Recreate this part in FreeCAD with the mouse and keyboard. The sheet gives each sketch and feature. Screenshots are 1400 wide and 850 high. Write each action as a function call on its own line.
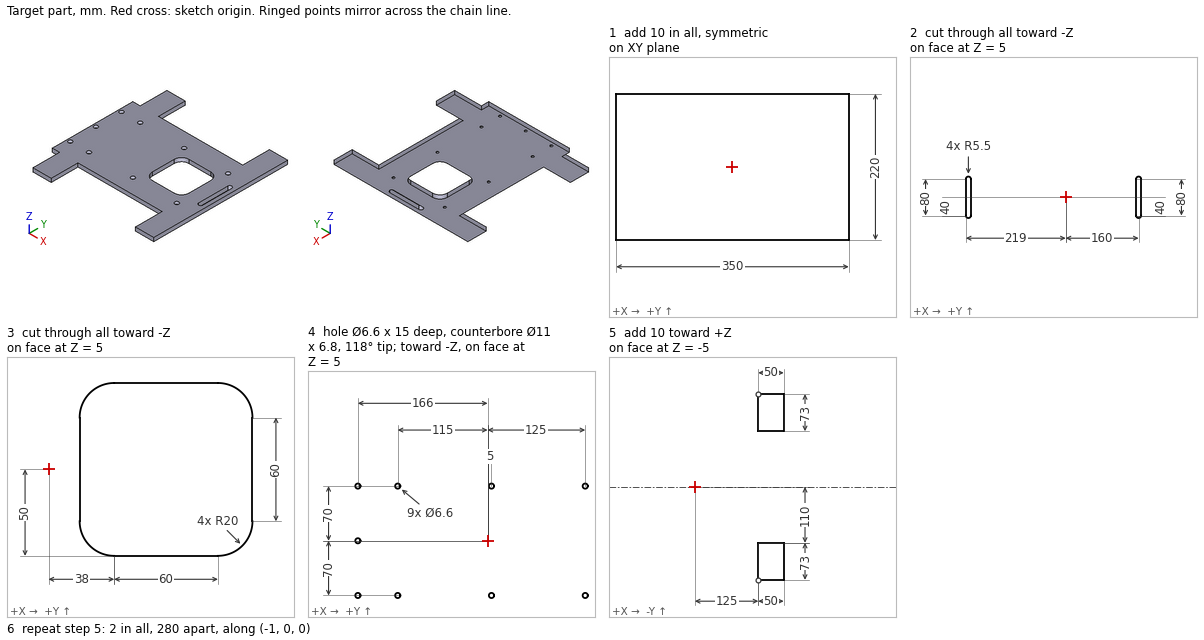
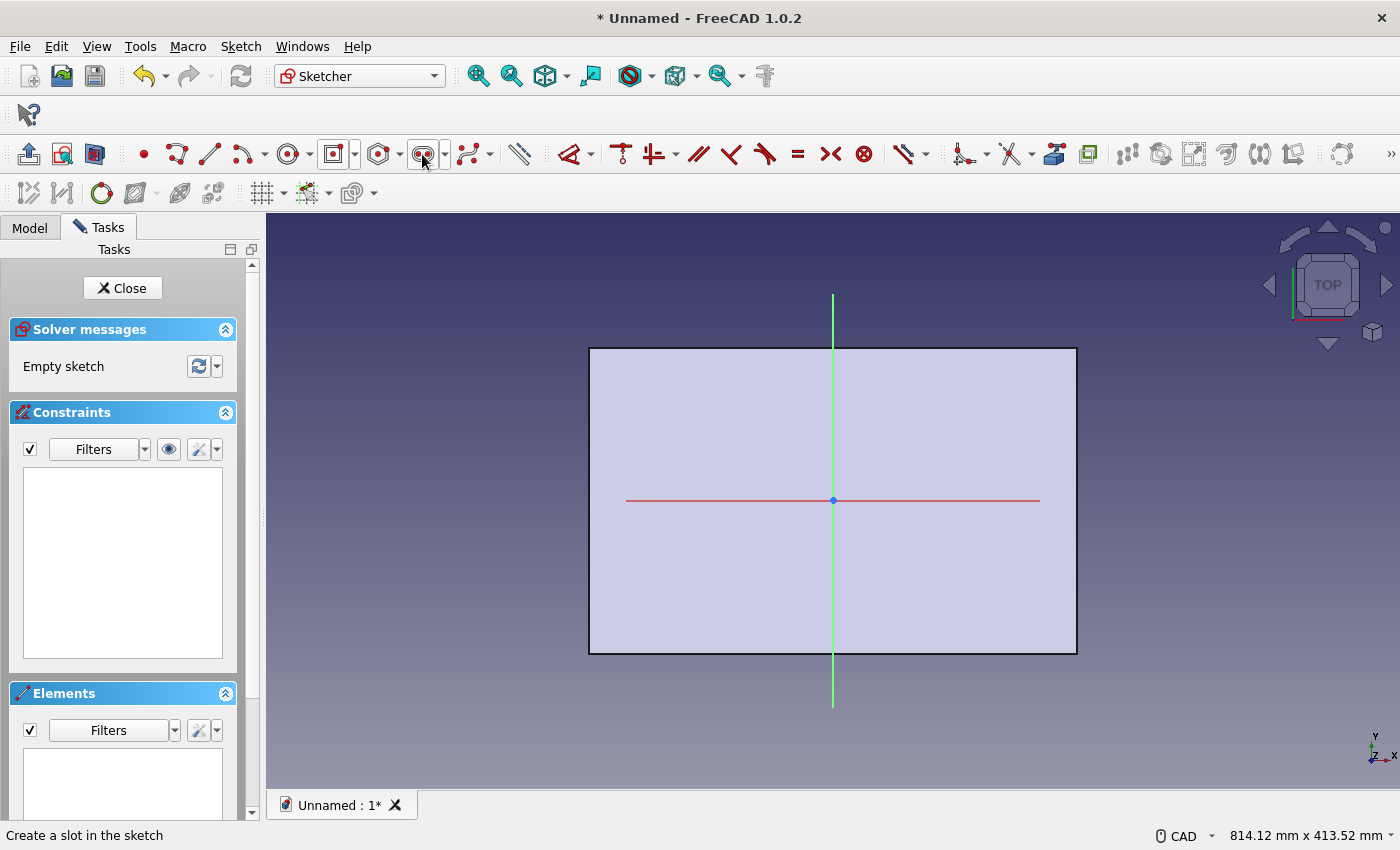
scroll(536, 557, up, 6)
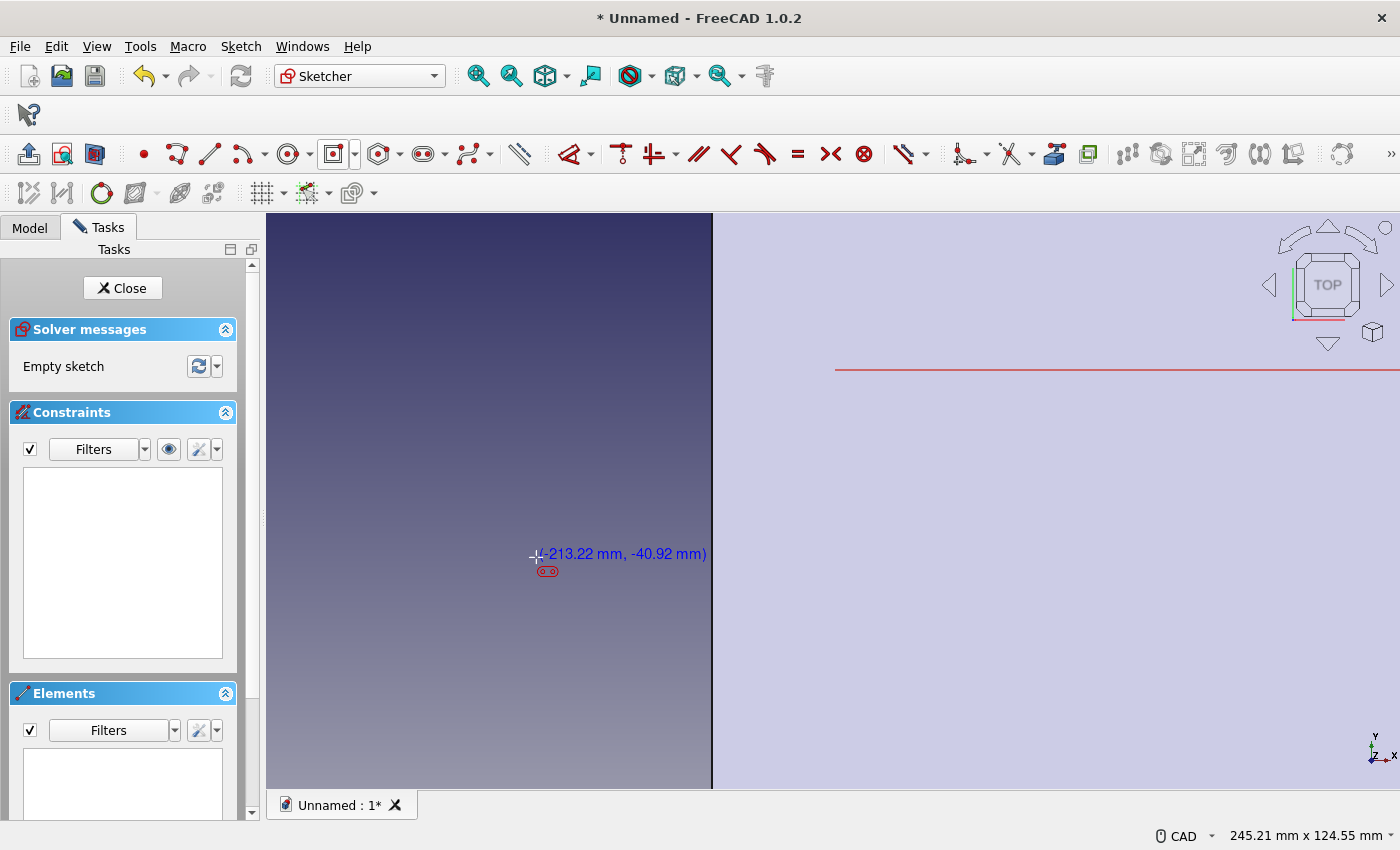
click(534, 555)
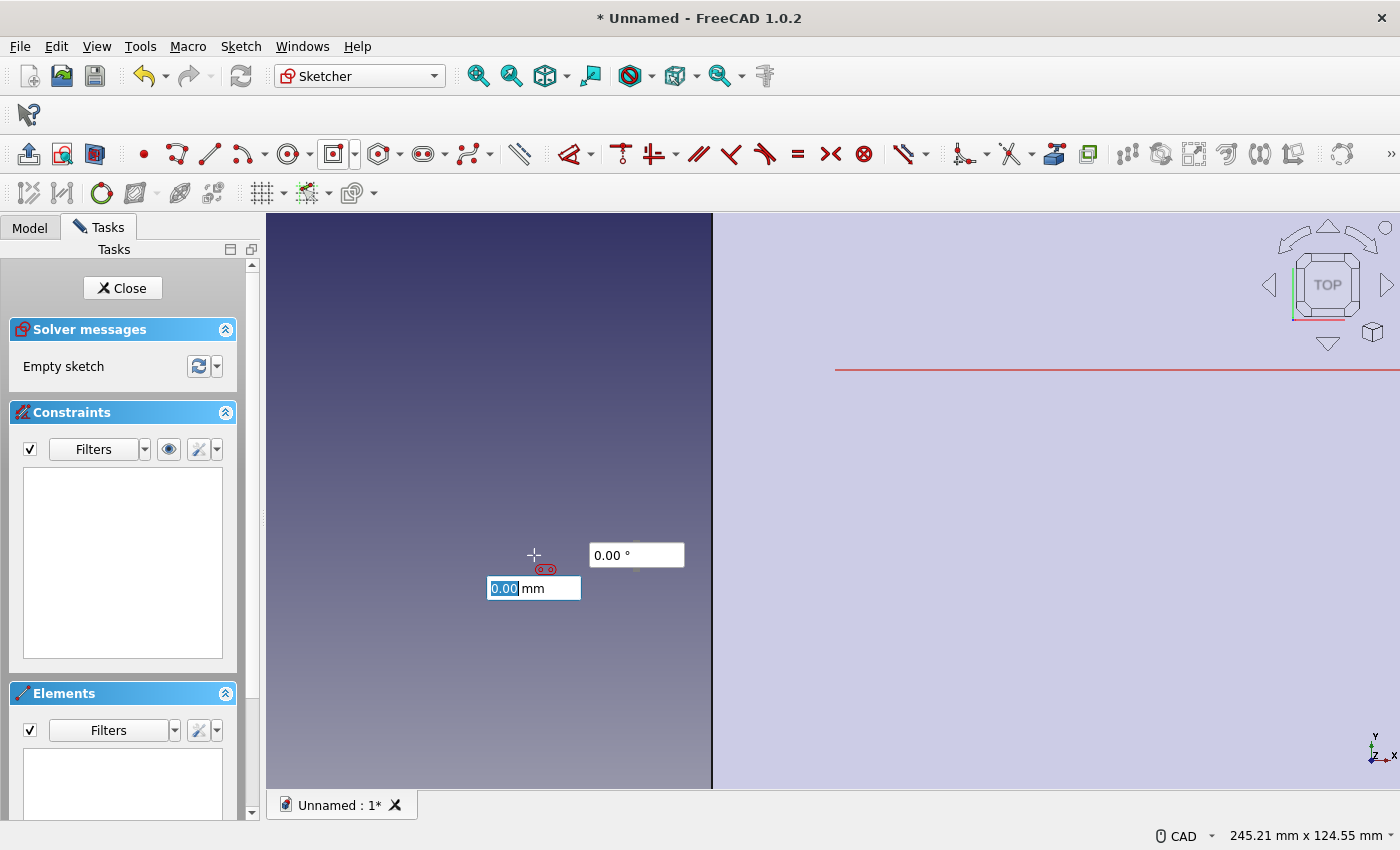
scroll(396, 577, down, 5)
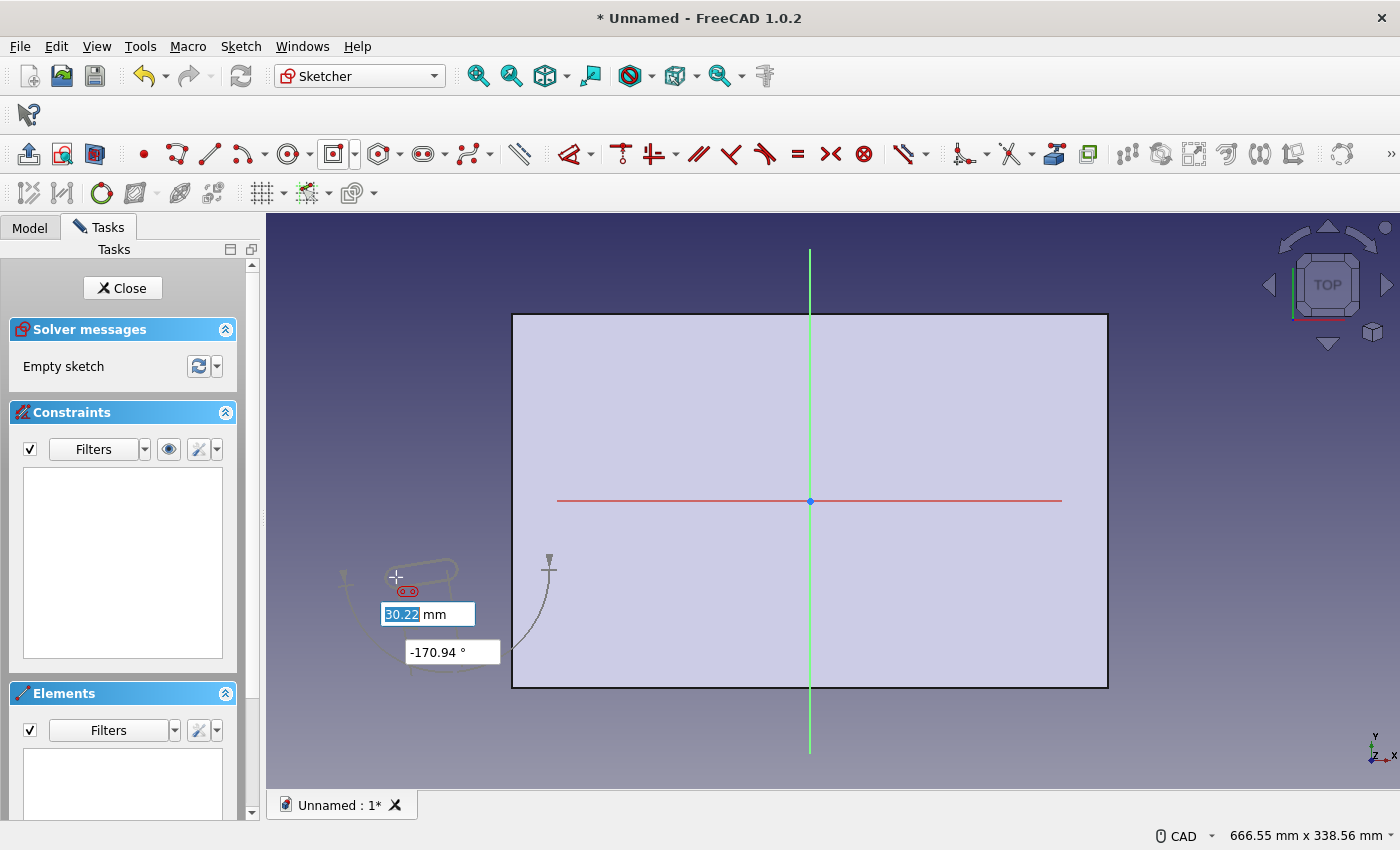
click(447, 433)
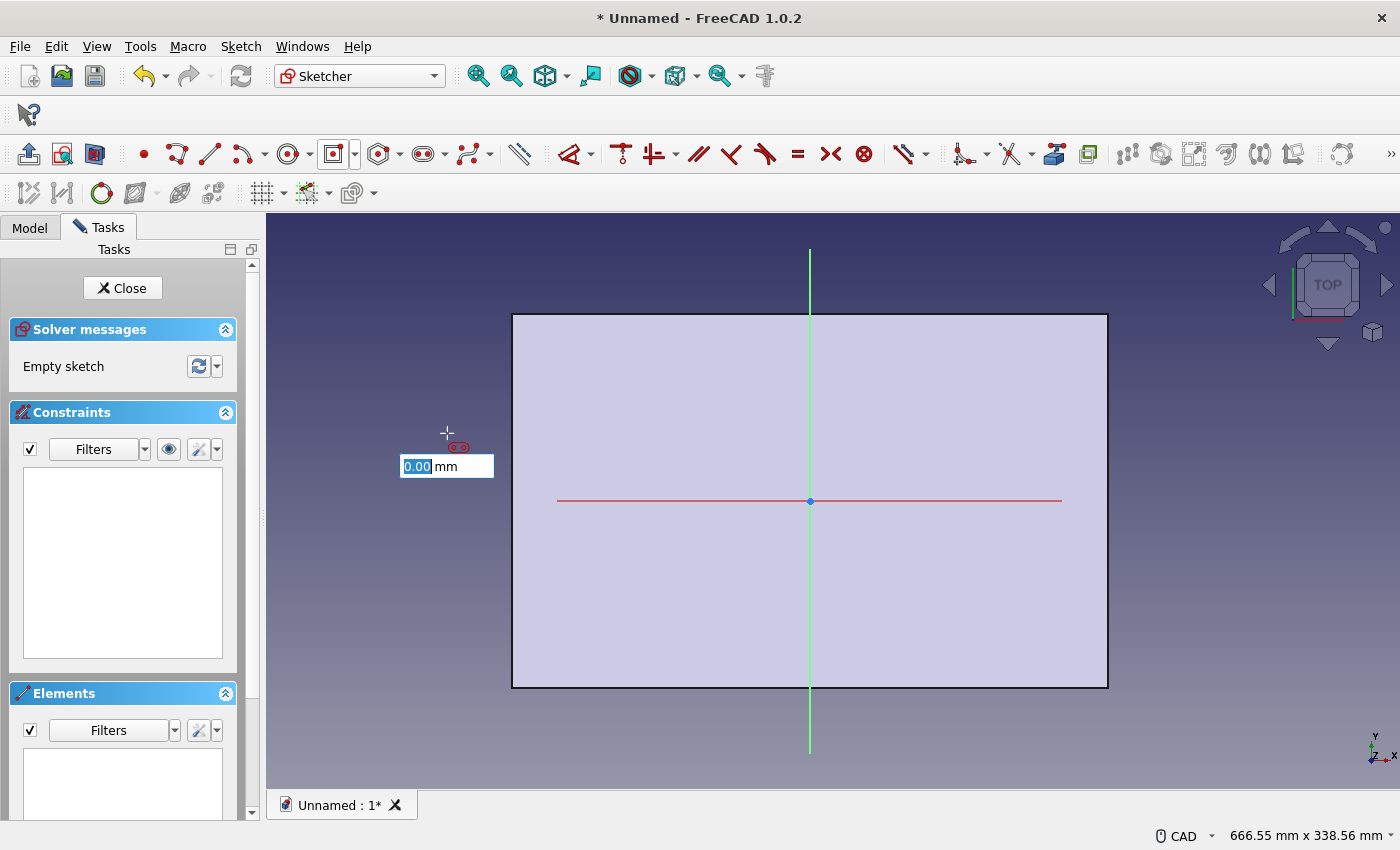
scroll(456, 522, up, 3)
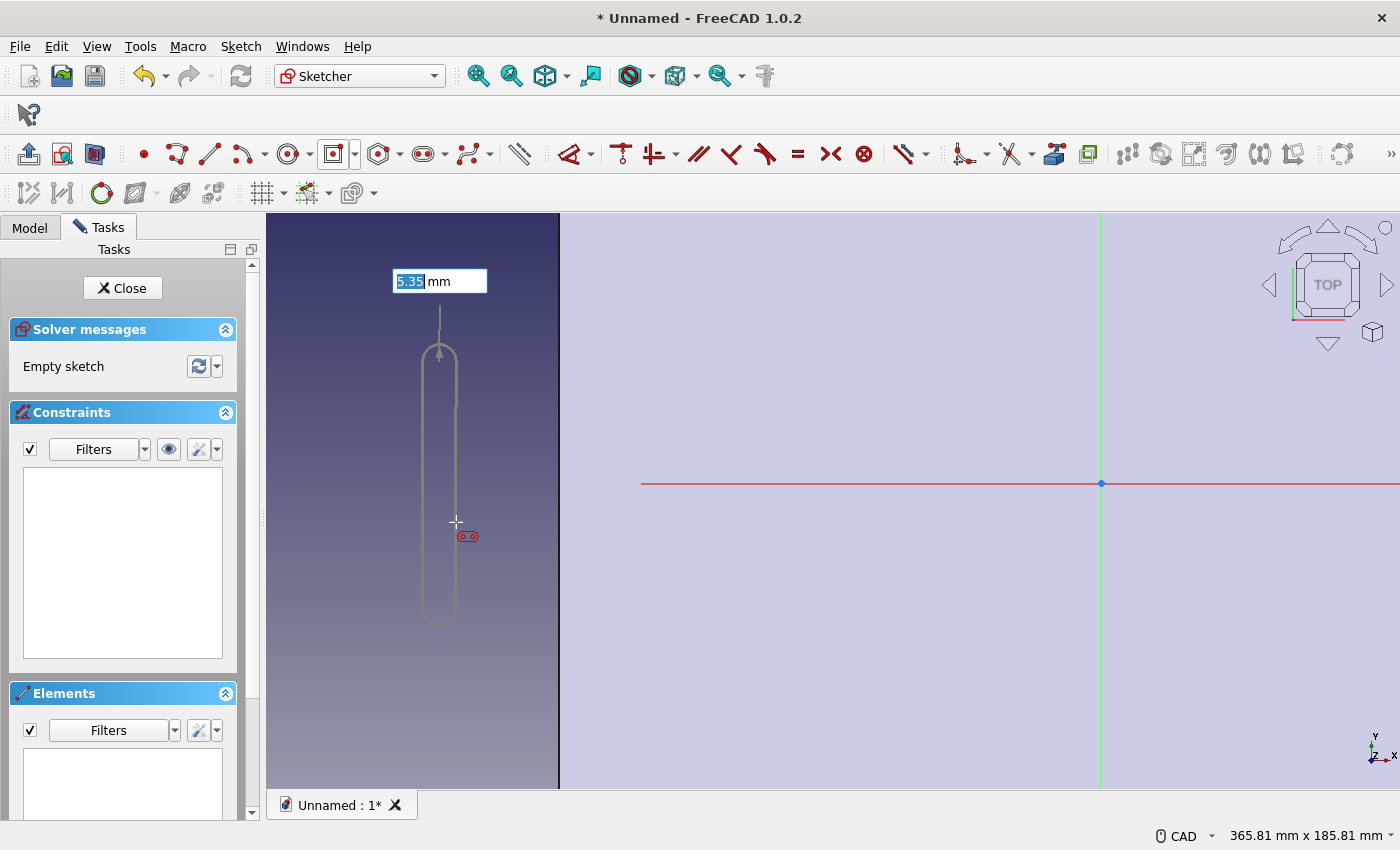
click(456, 521)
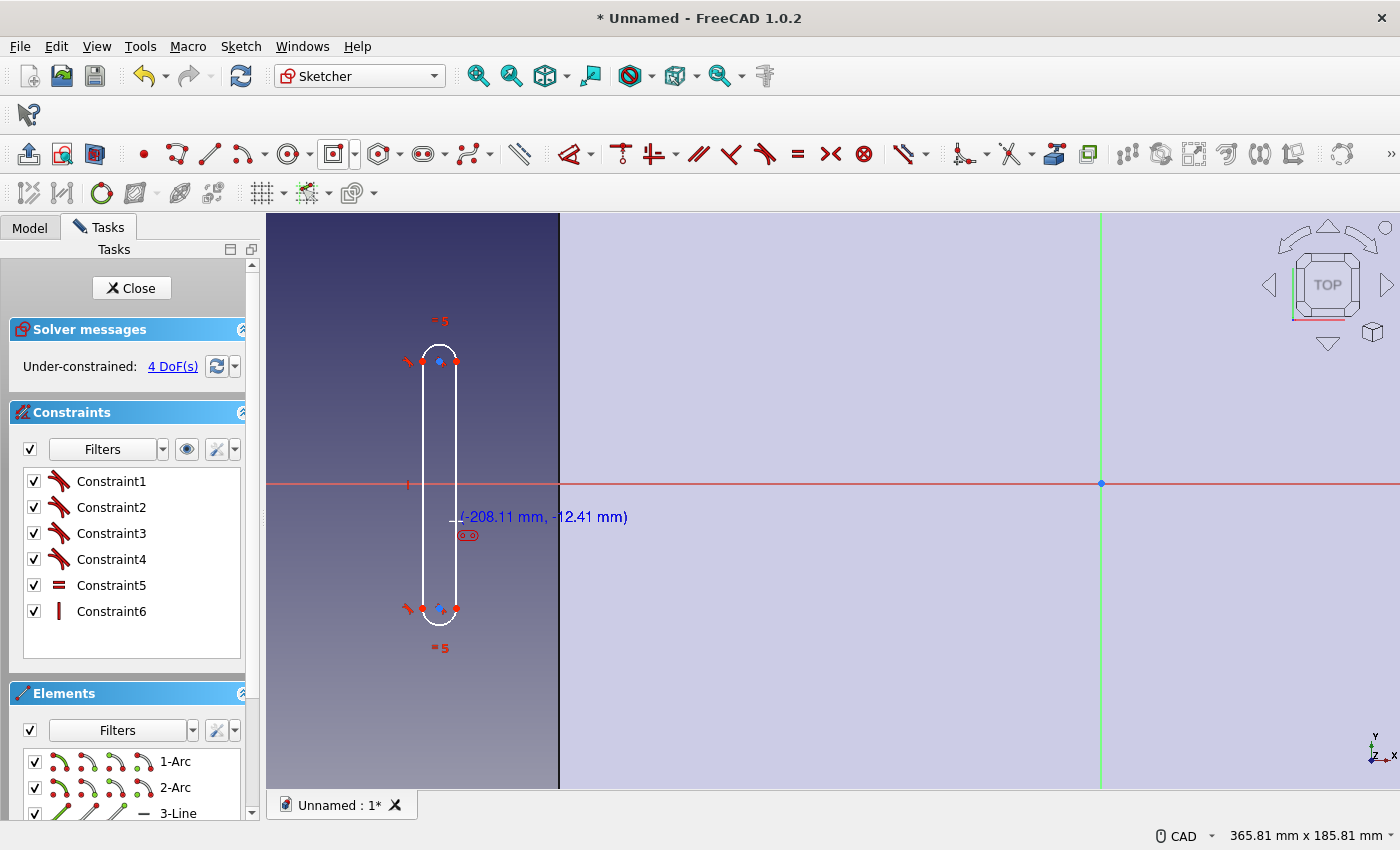
scroll(456, 522, down, 3)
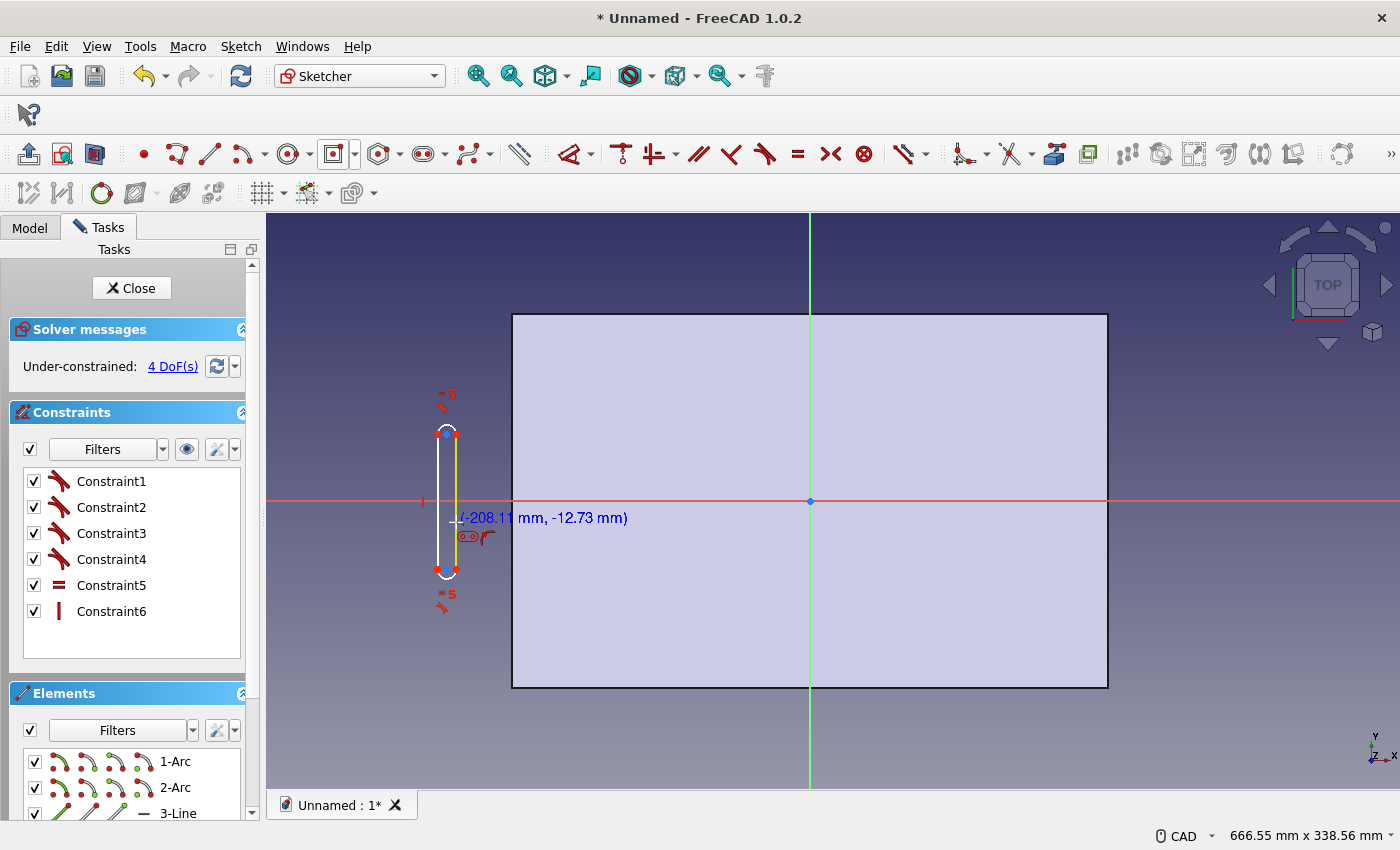
scroll(1082, 569, up, 5)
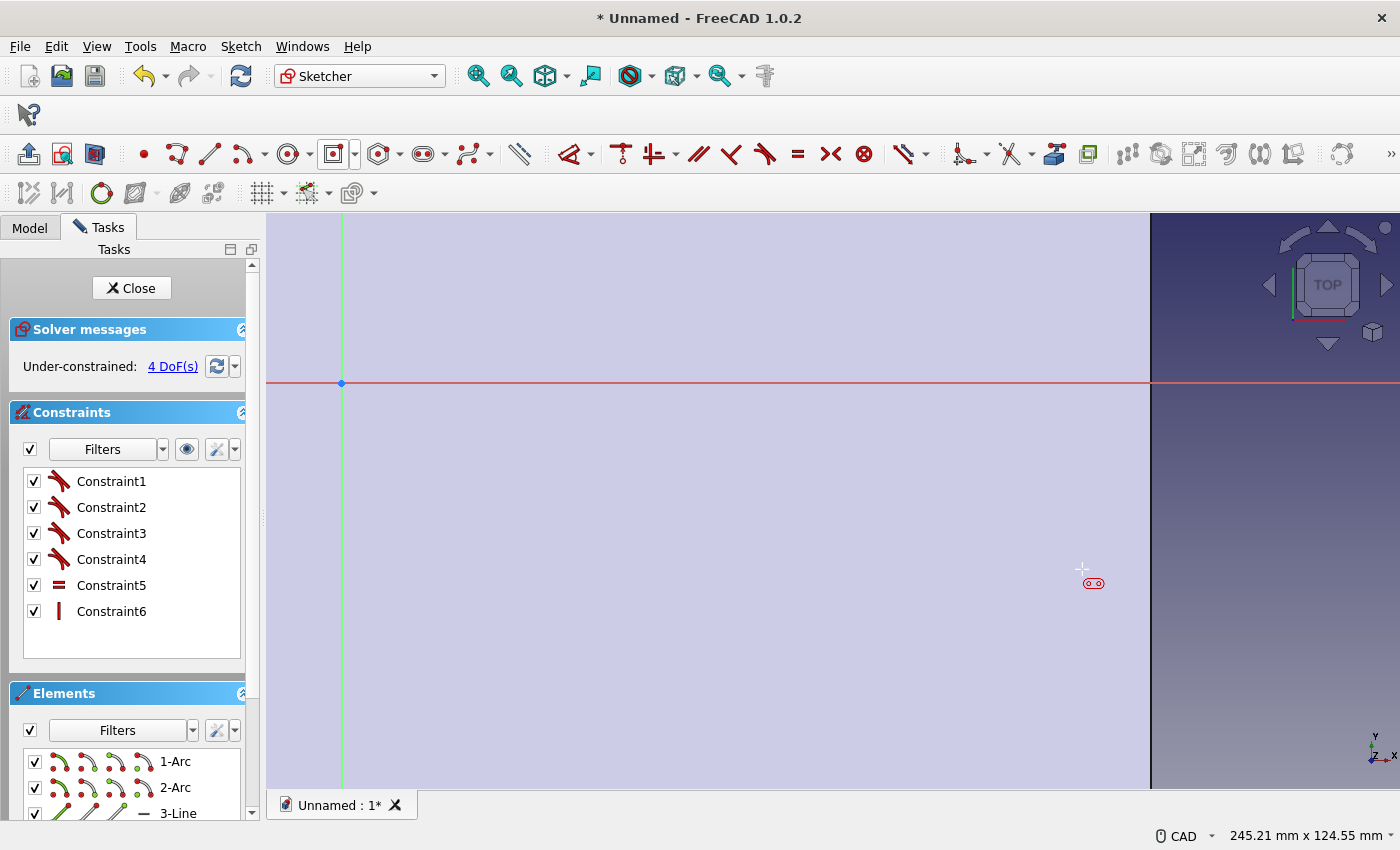
click(1082, 568)